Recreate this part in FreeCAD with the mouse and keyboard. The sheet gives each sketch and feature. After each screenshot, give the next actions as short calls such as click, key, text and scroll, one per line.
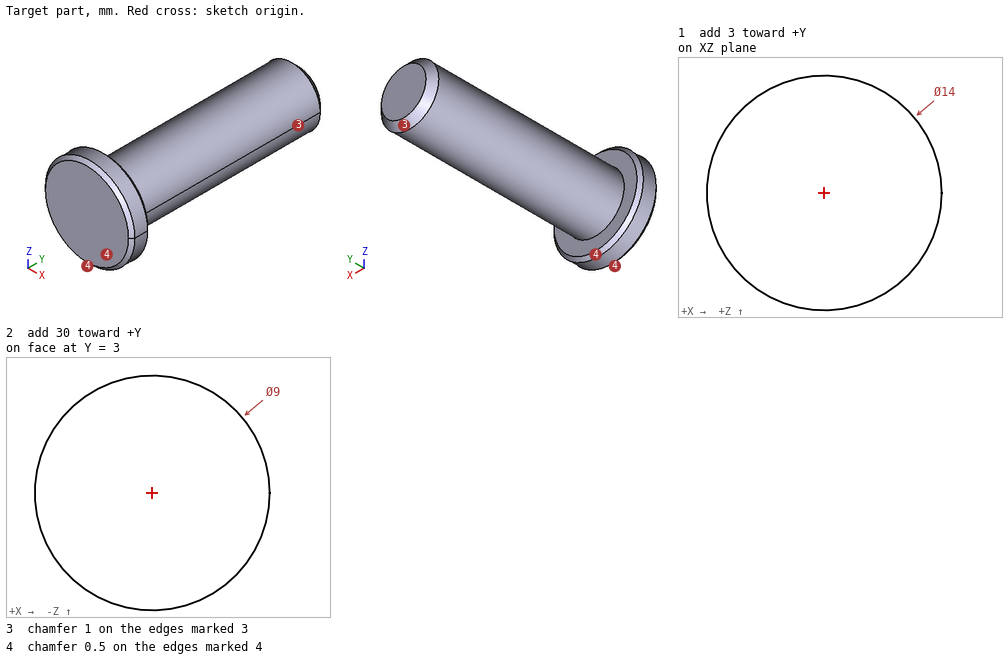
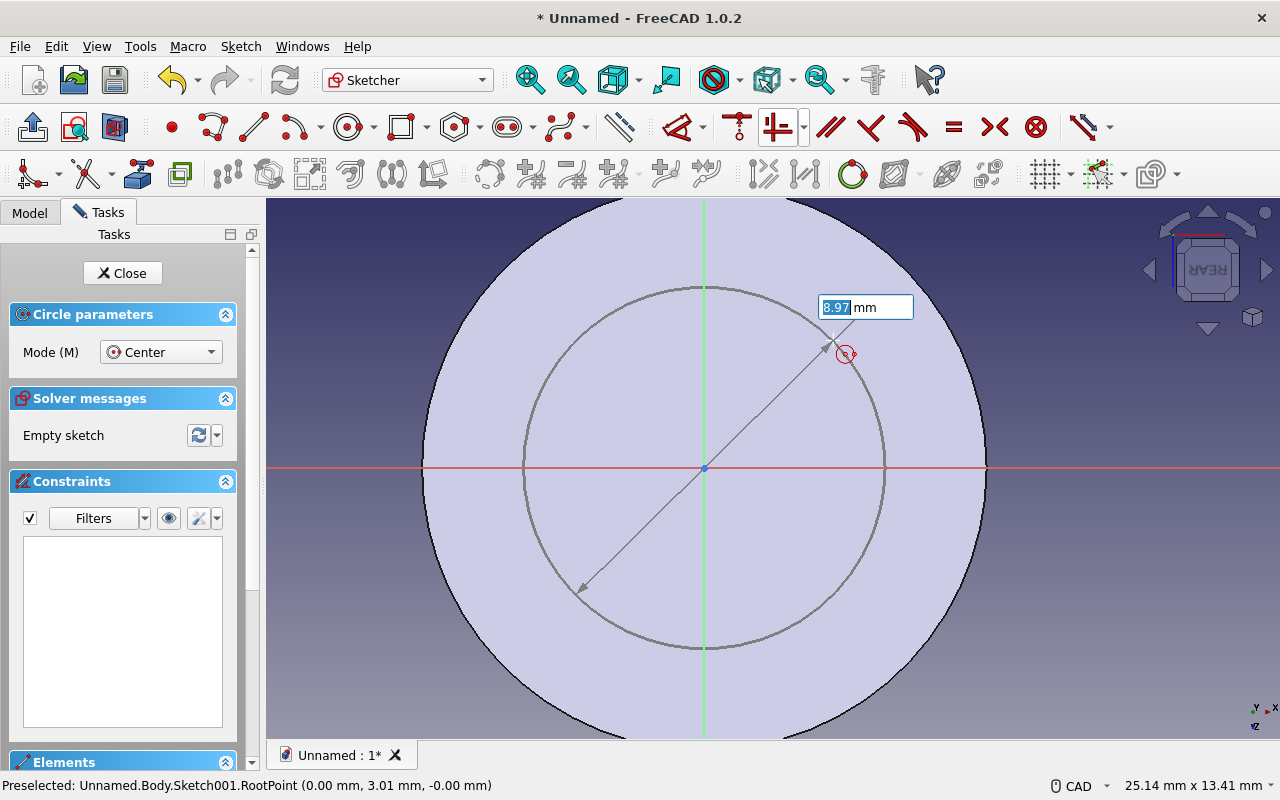
text(9)
key(Return)
key(Escape)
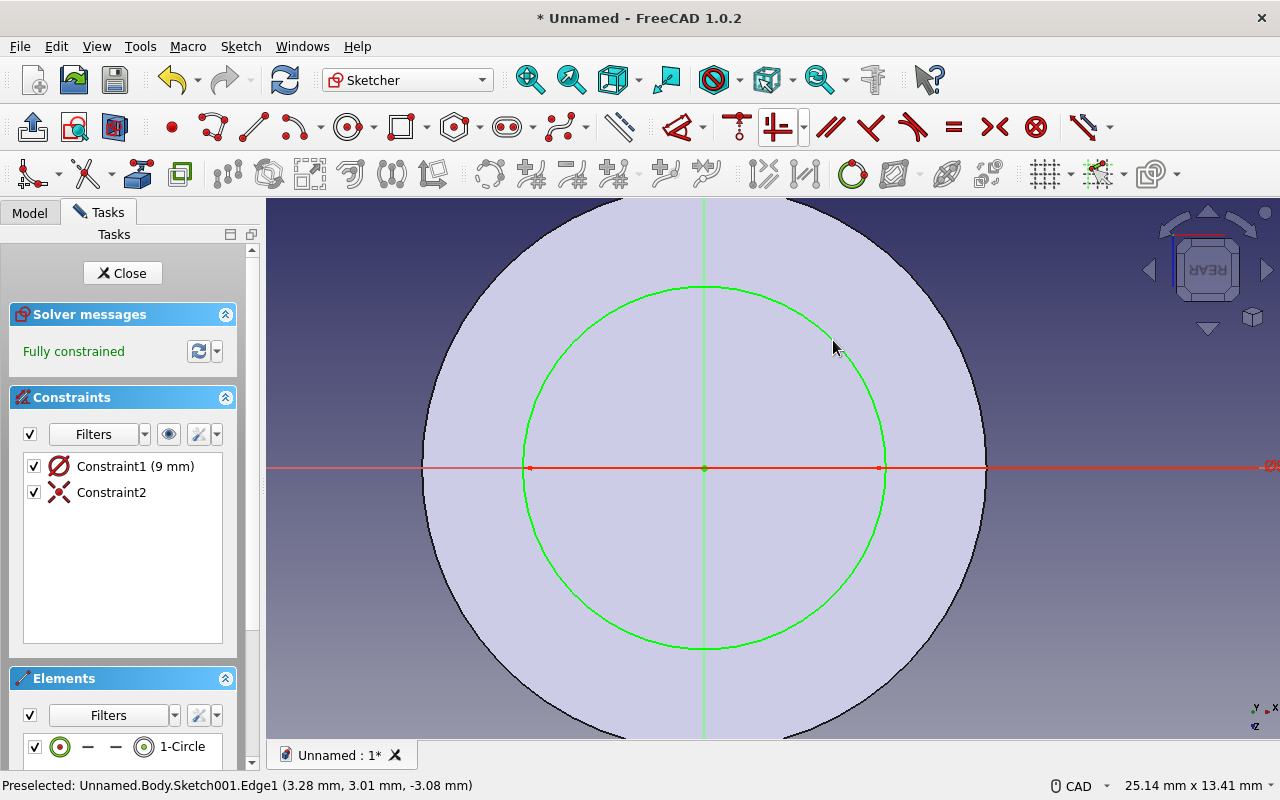
click(123, 273)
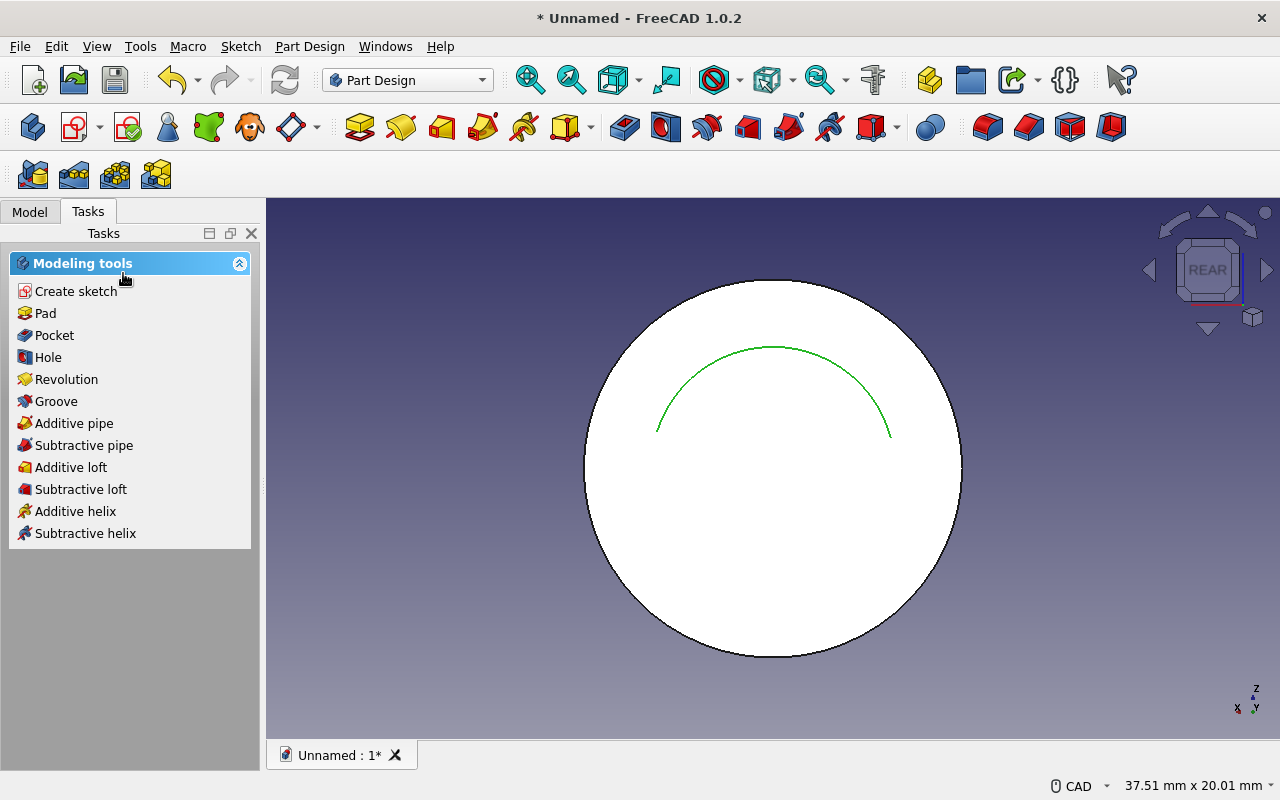
click(360, 128)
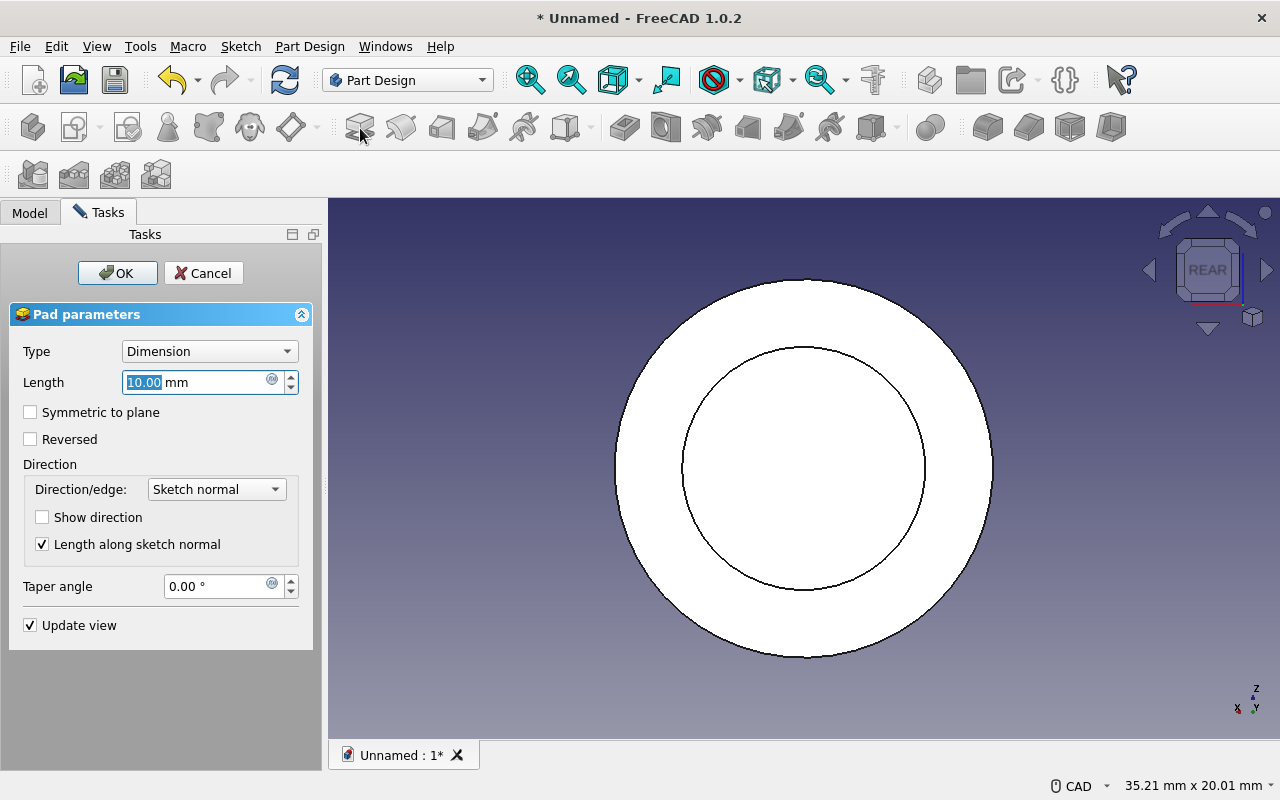
text(30)
key(Tab)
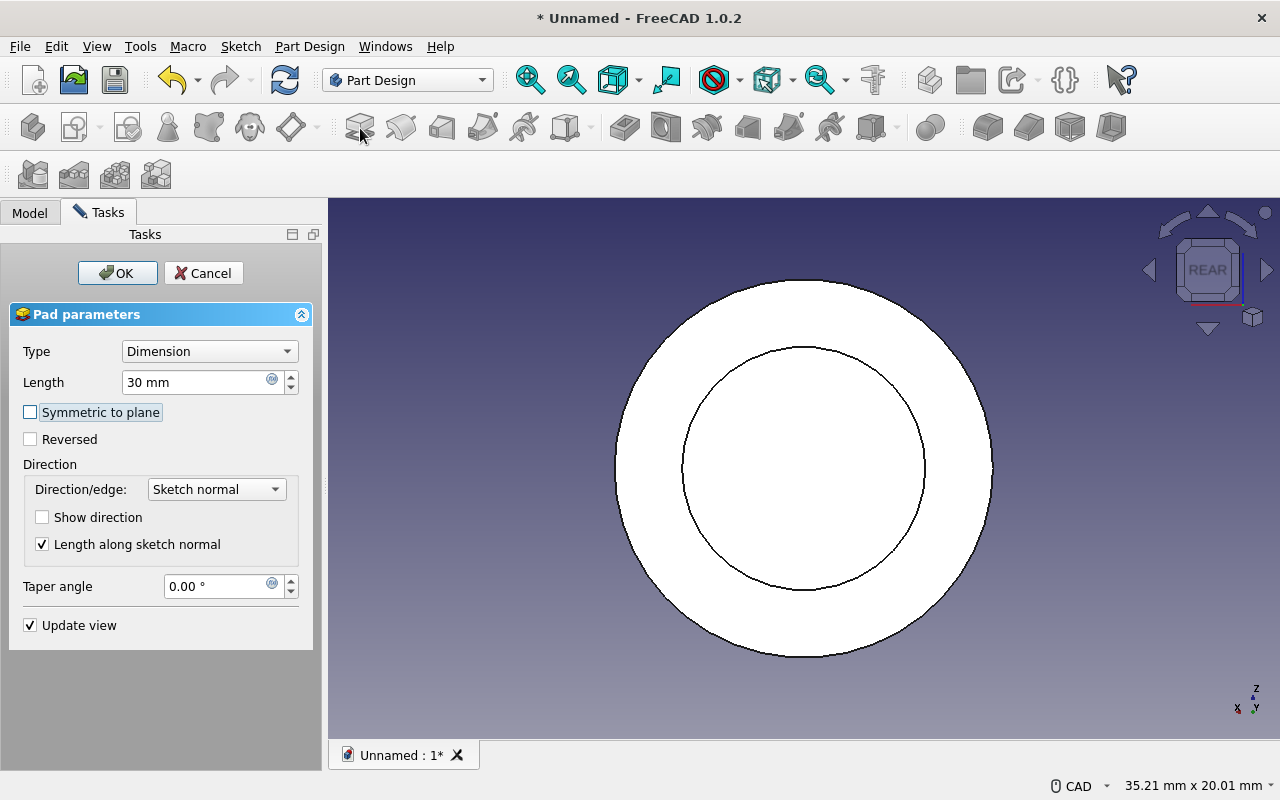
click(118, 273)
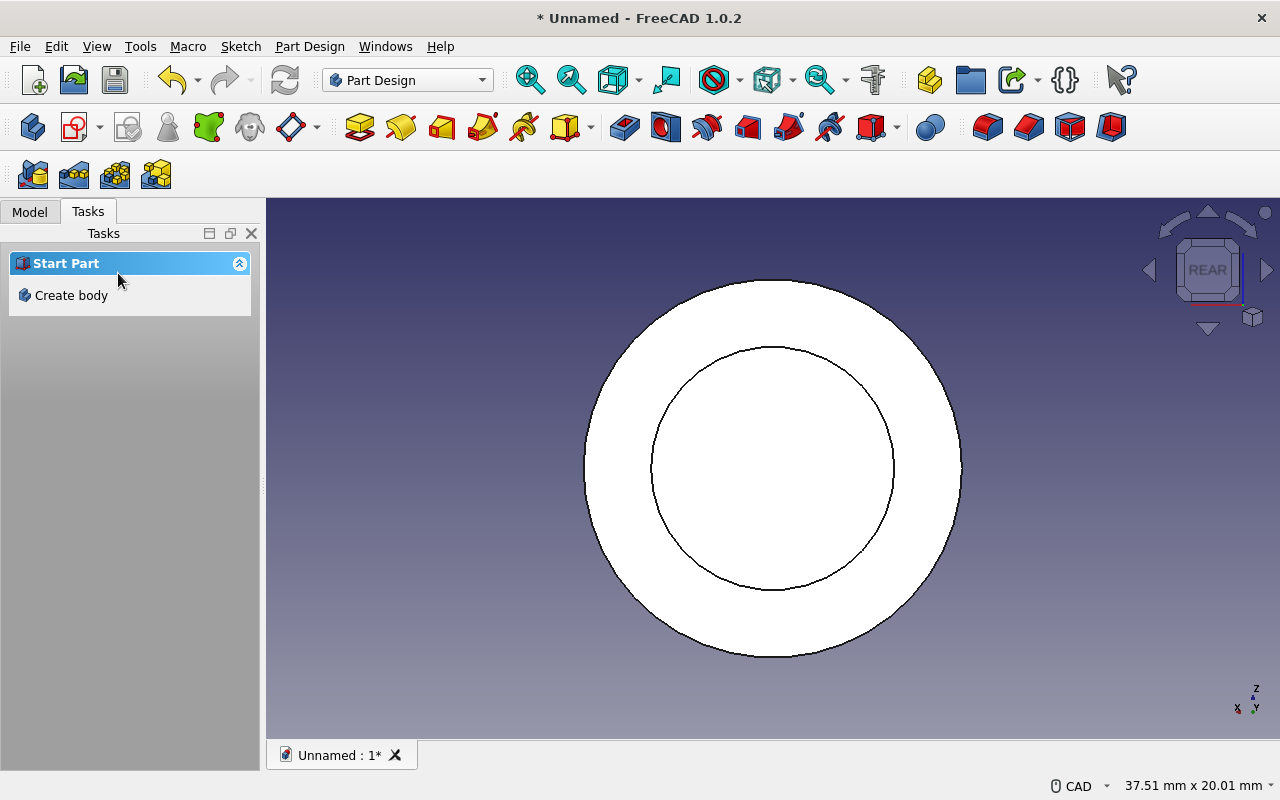
click(894, 468)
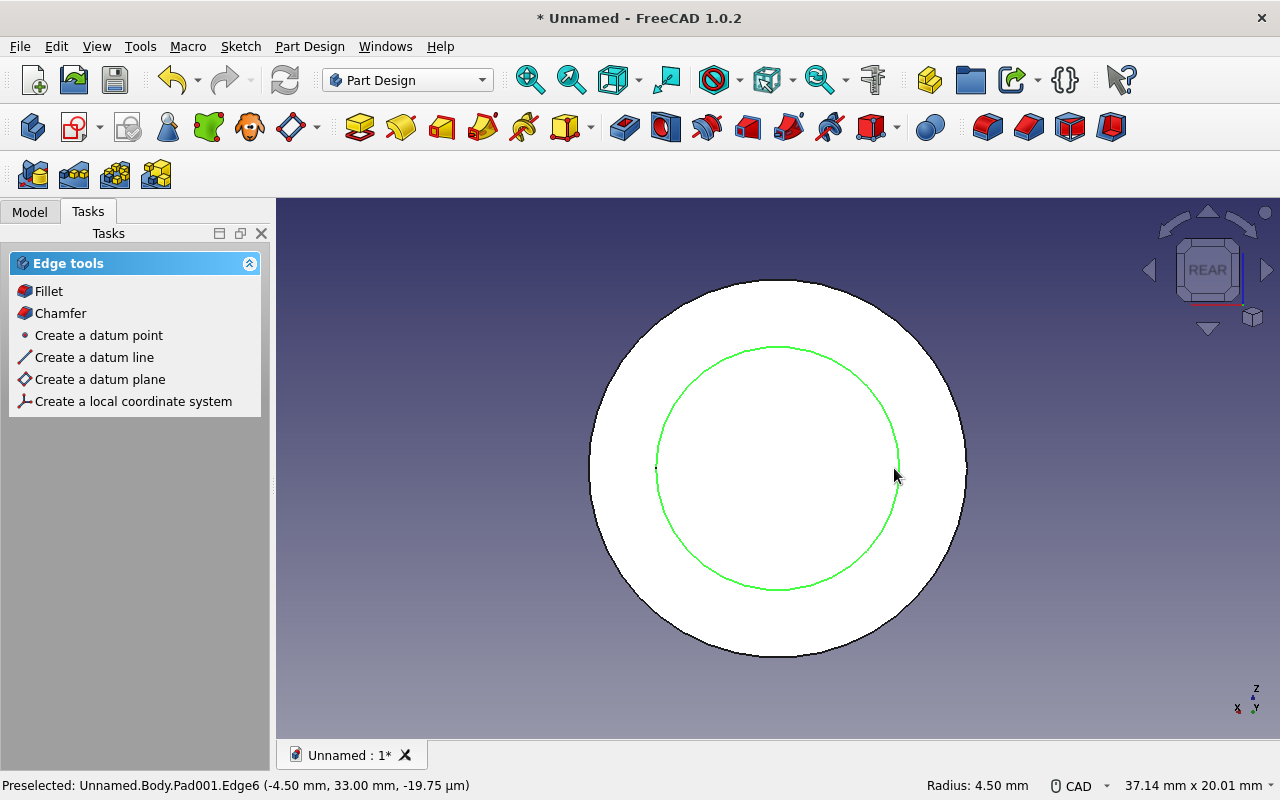
click(1029, 128)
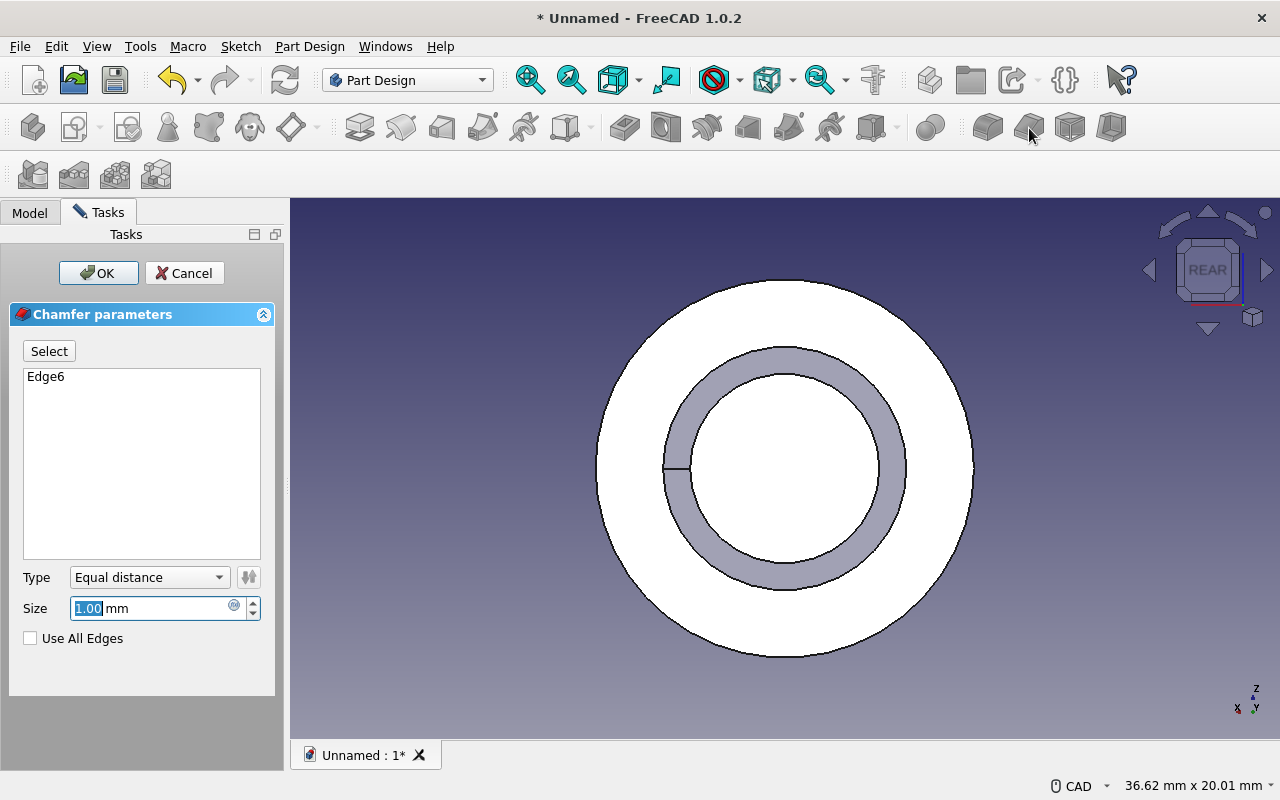
text(1)
key(Tab)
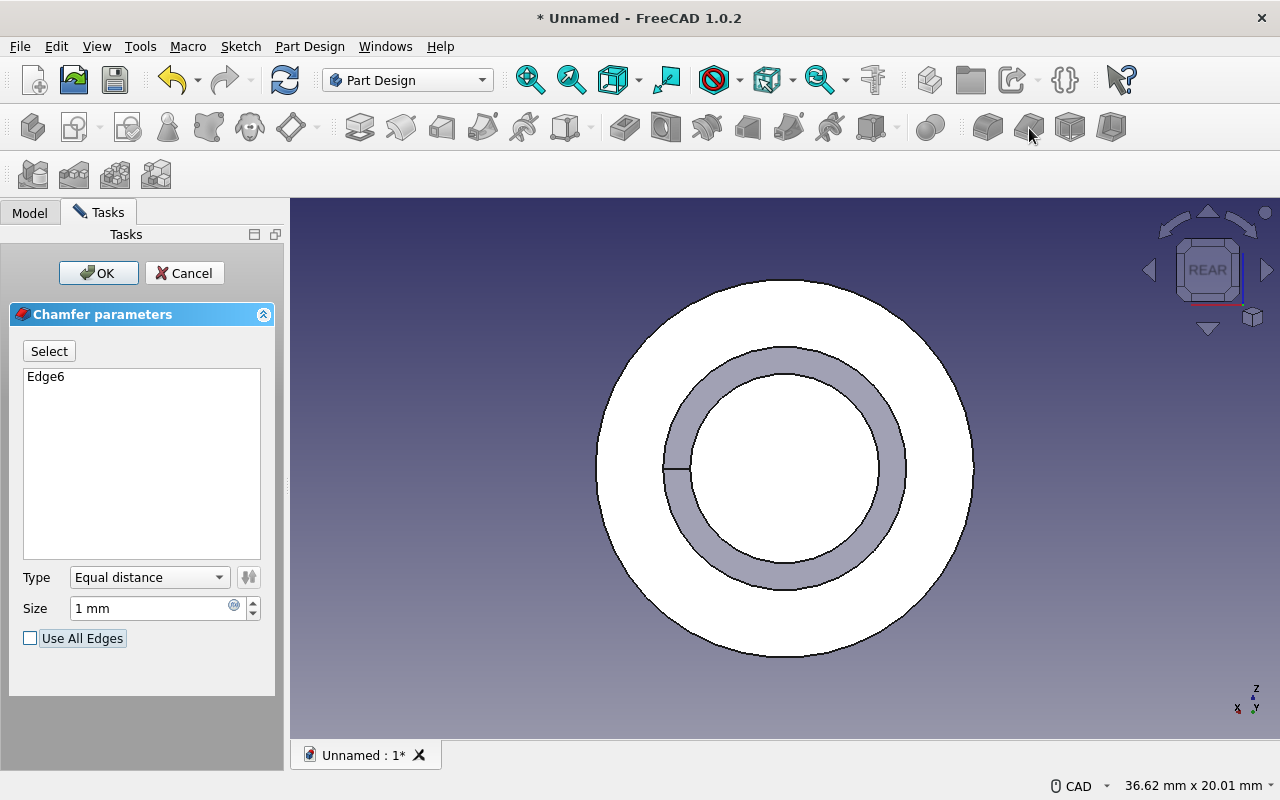
click(99, 273)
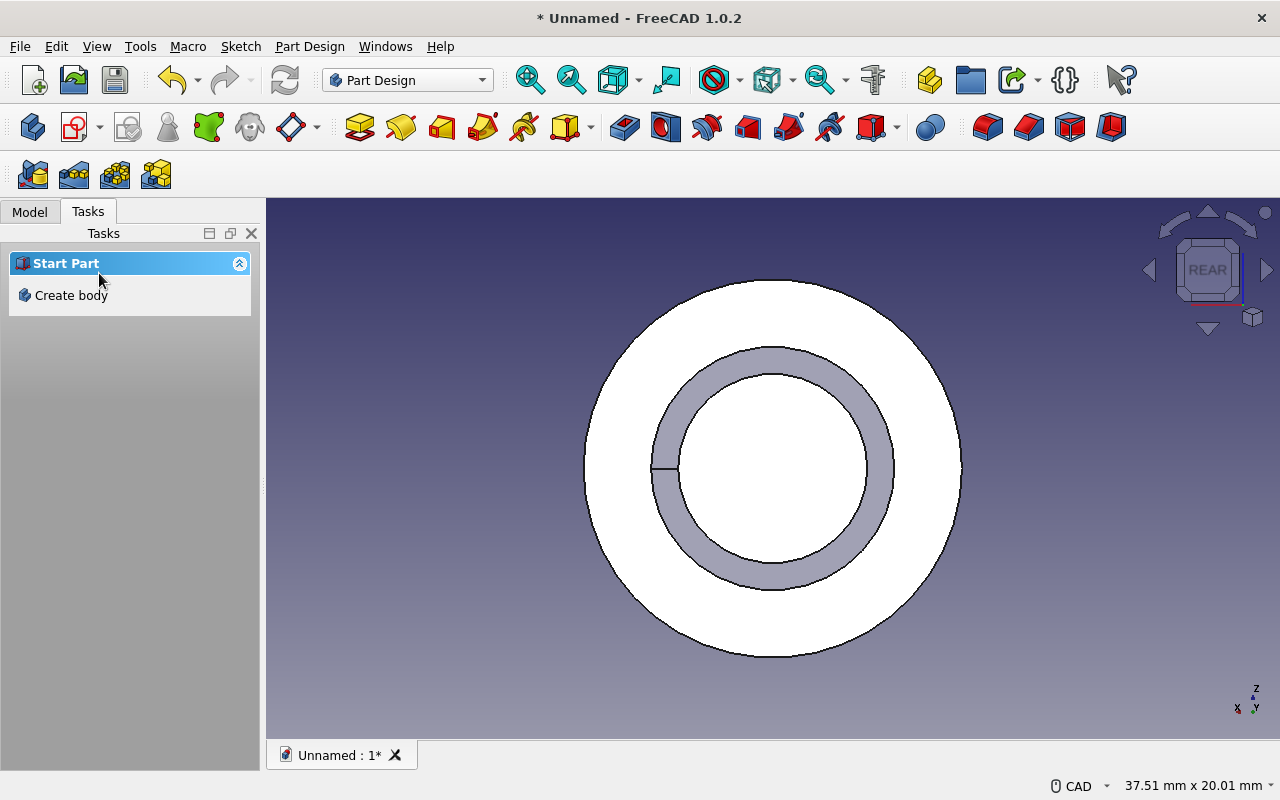
click(962, 468)